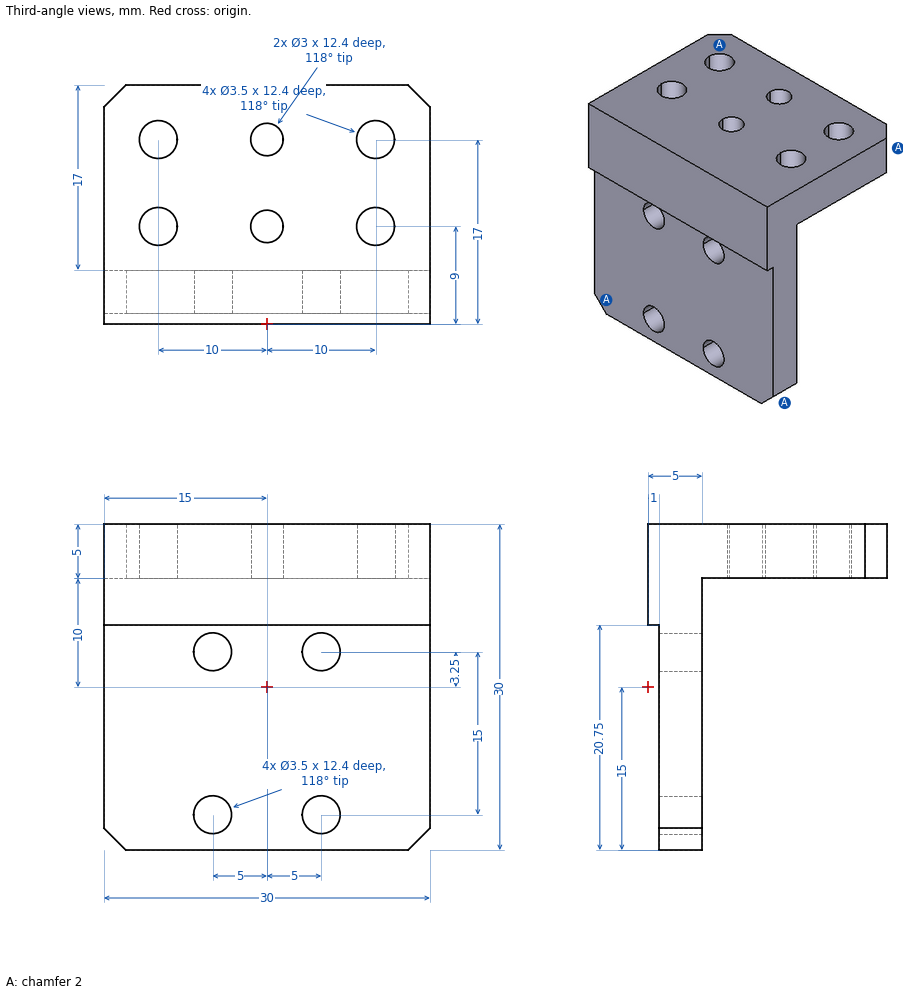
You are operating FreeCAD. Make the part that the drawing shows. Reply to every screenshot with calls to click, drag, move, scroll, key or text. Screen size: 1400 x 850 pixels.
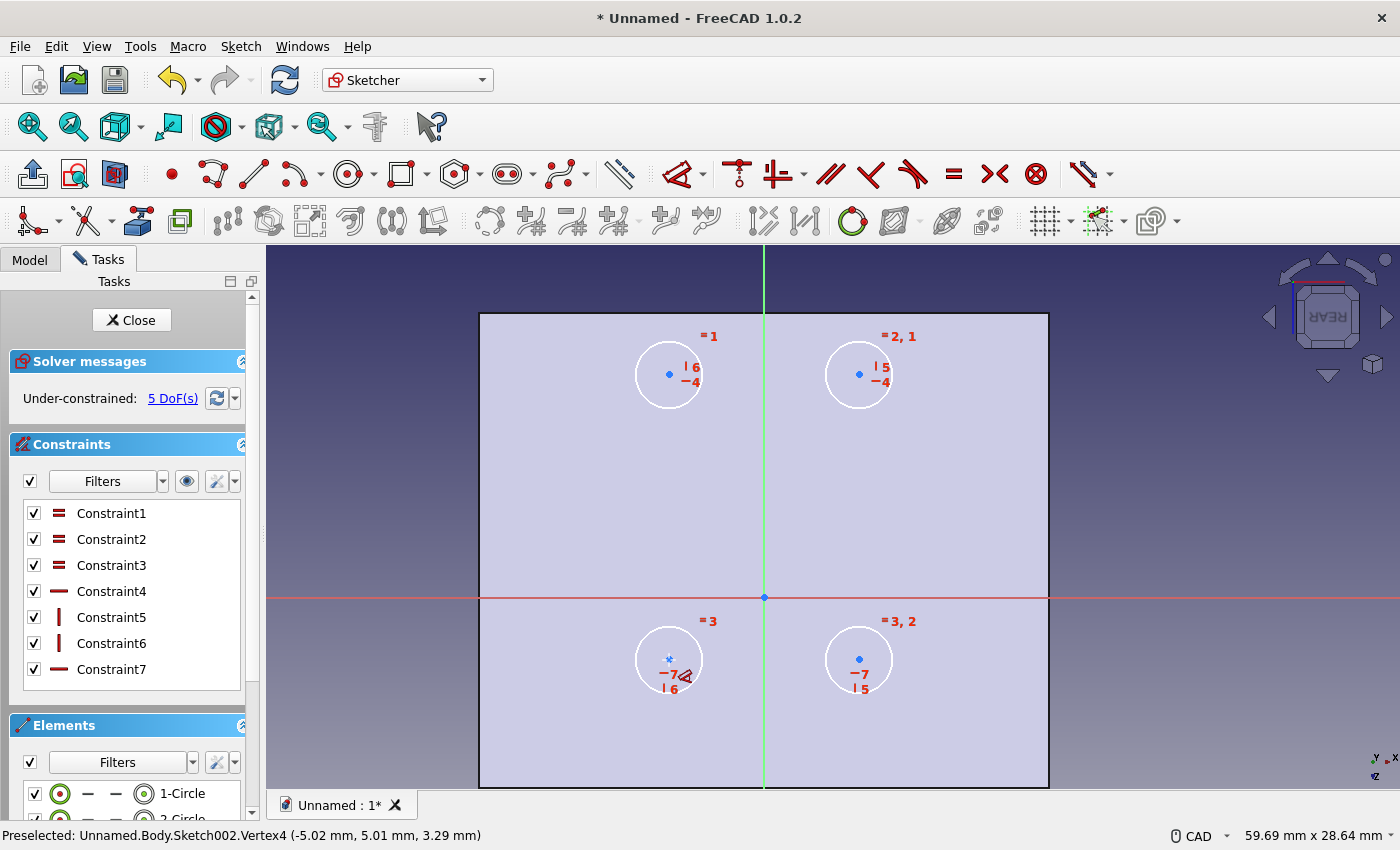
click(692, 351)
click(714, 328)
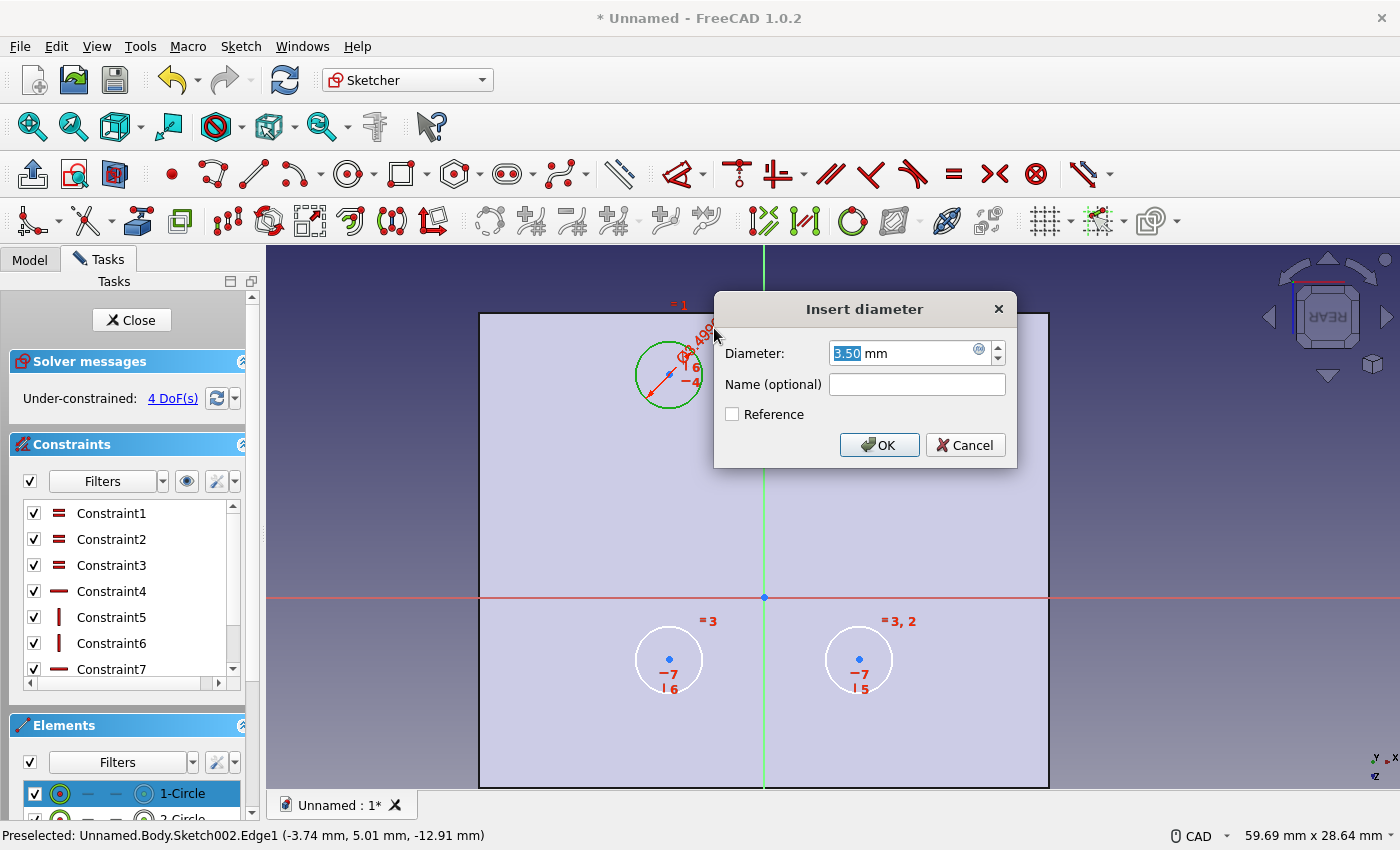
text(3.5)
key(Return)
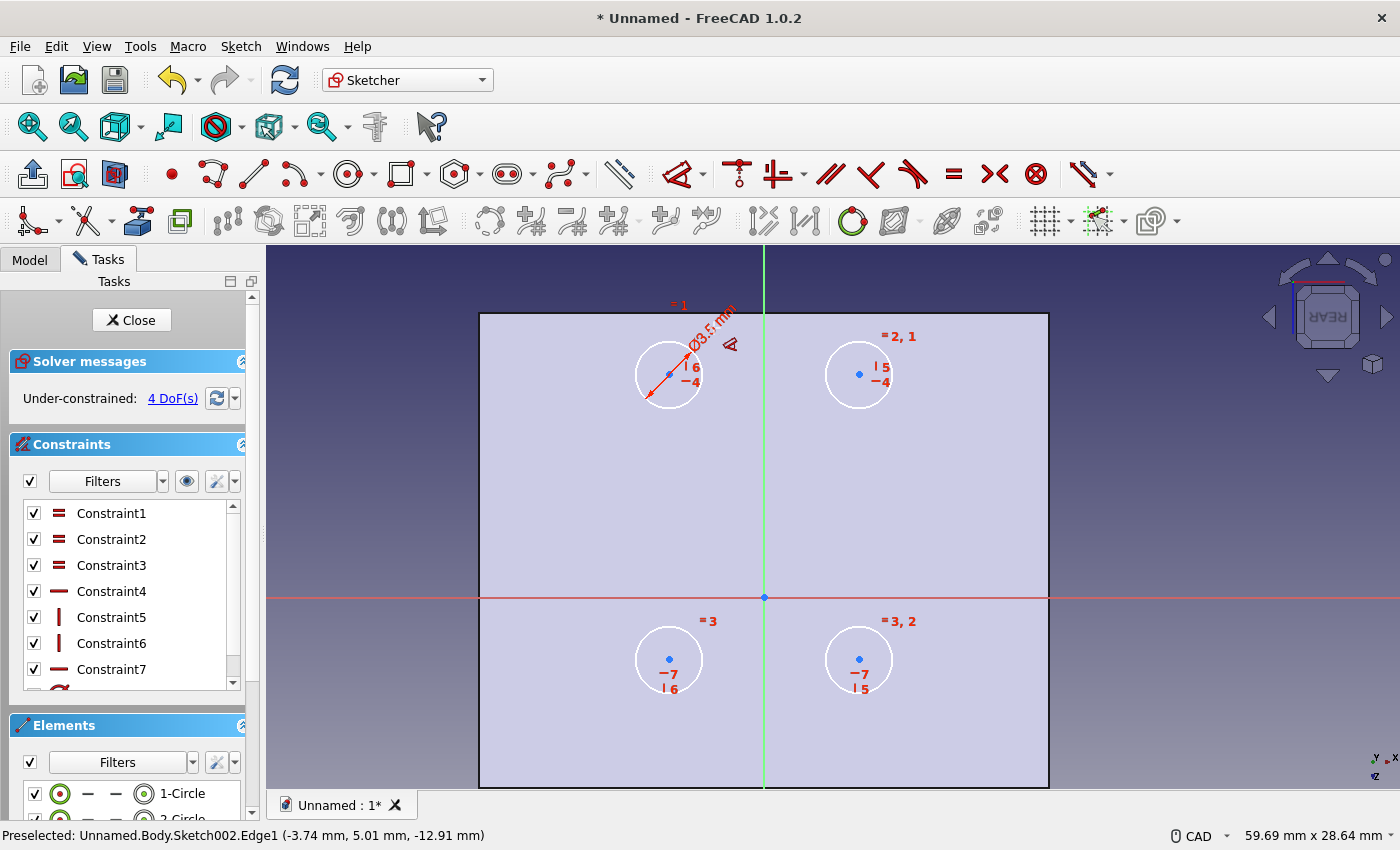
click(669, 375)
click(717, 632)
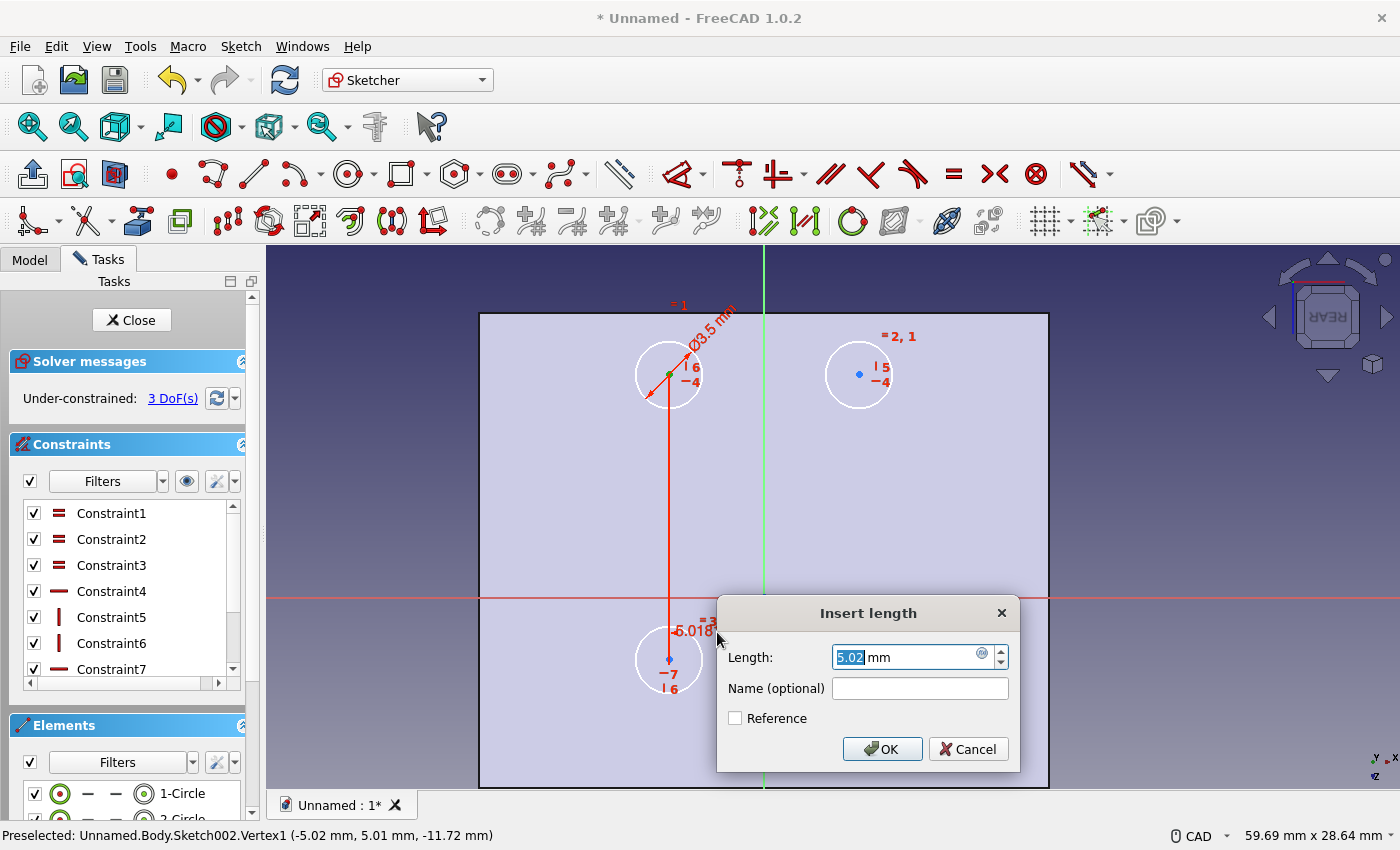
text(5)
key(Return)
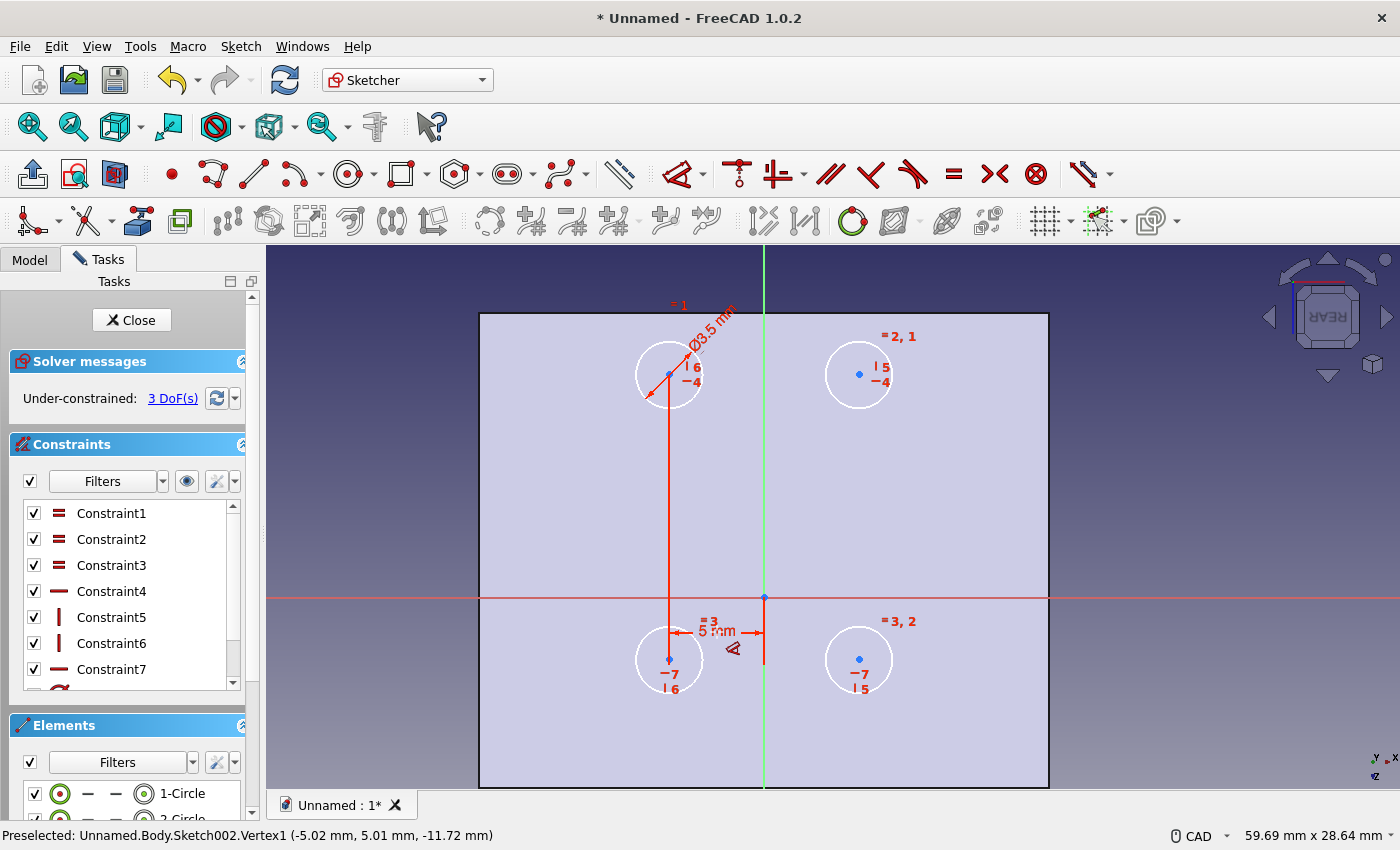
click(859, 375)
click(812, 341)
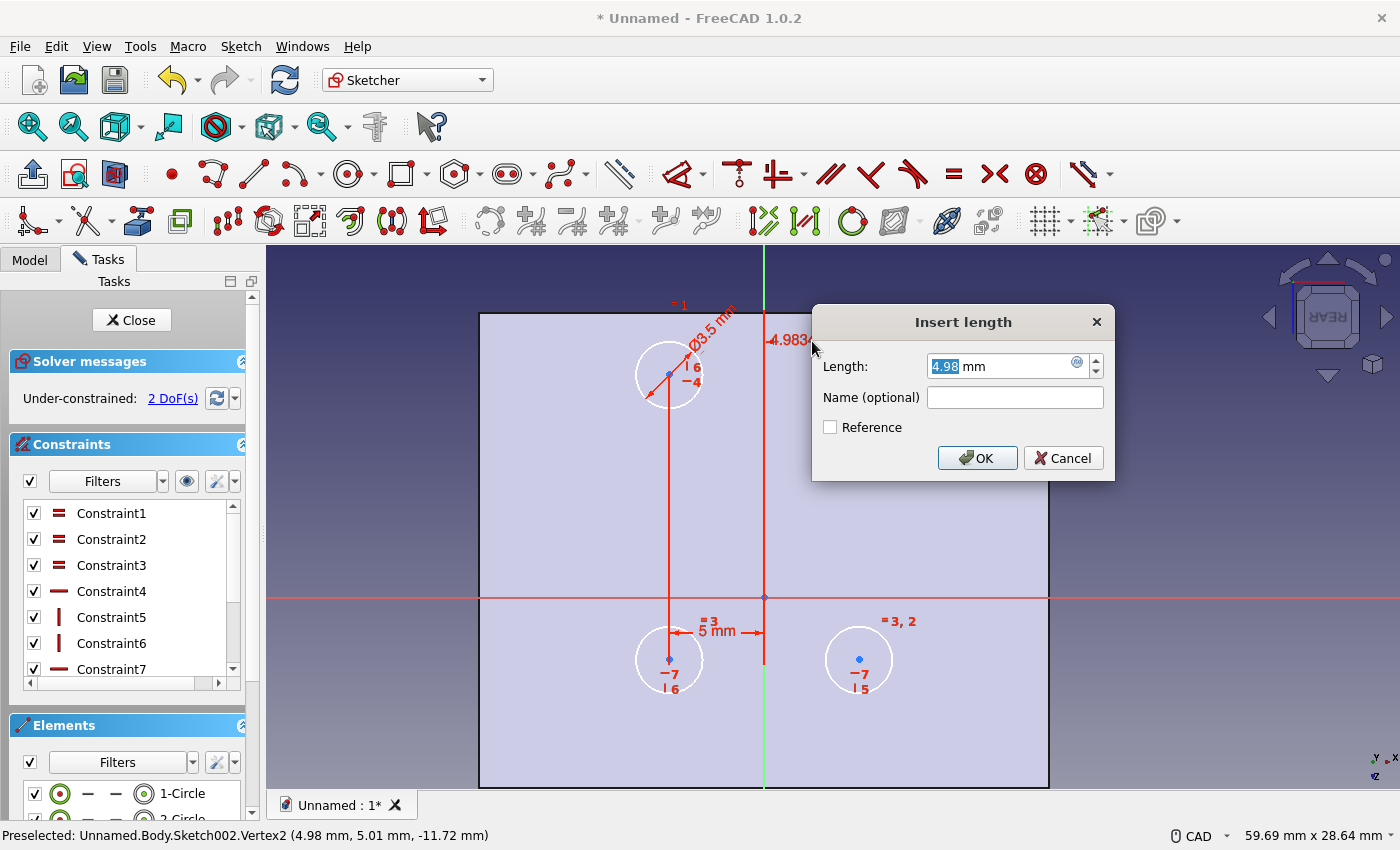
text(5)
key(Return)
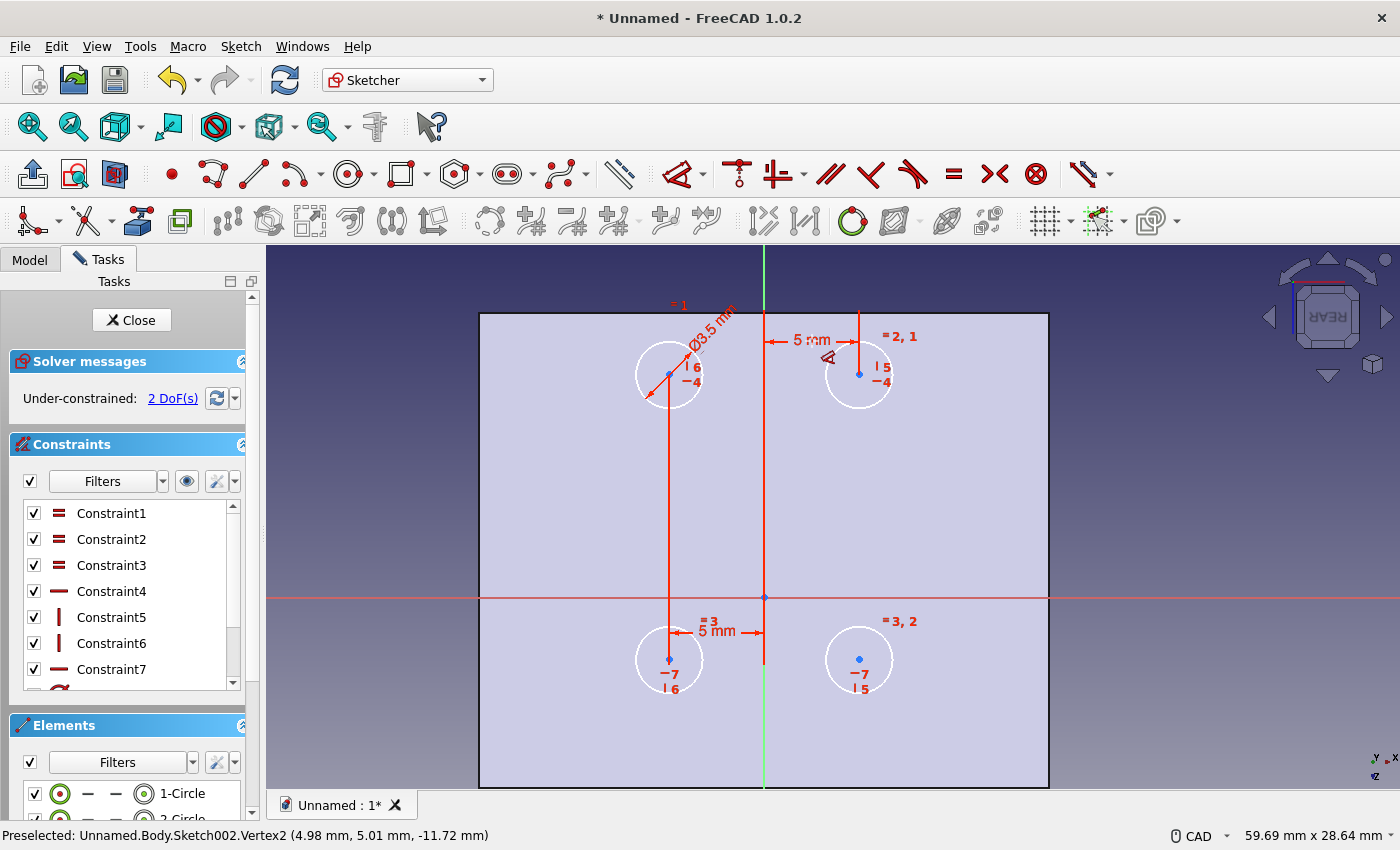
click(859, 375)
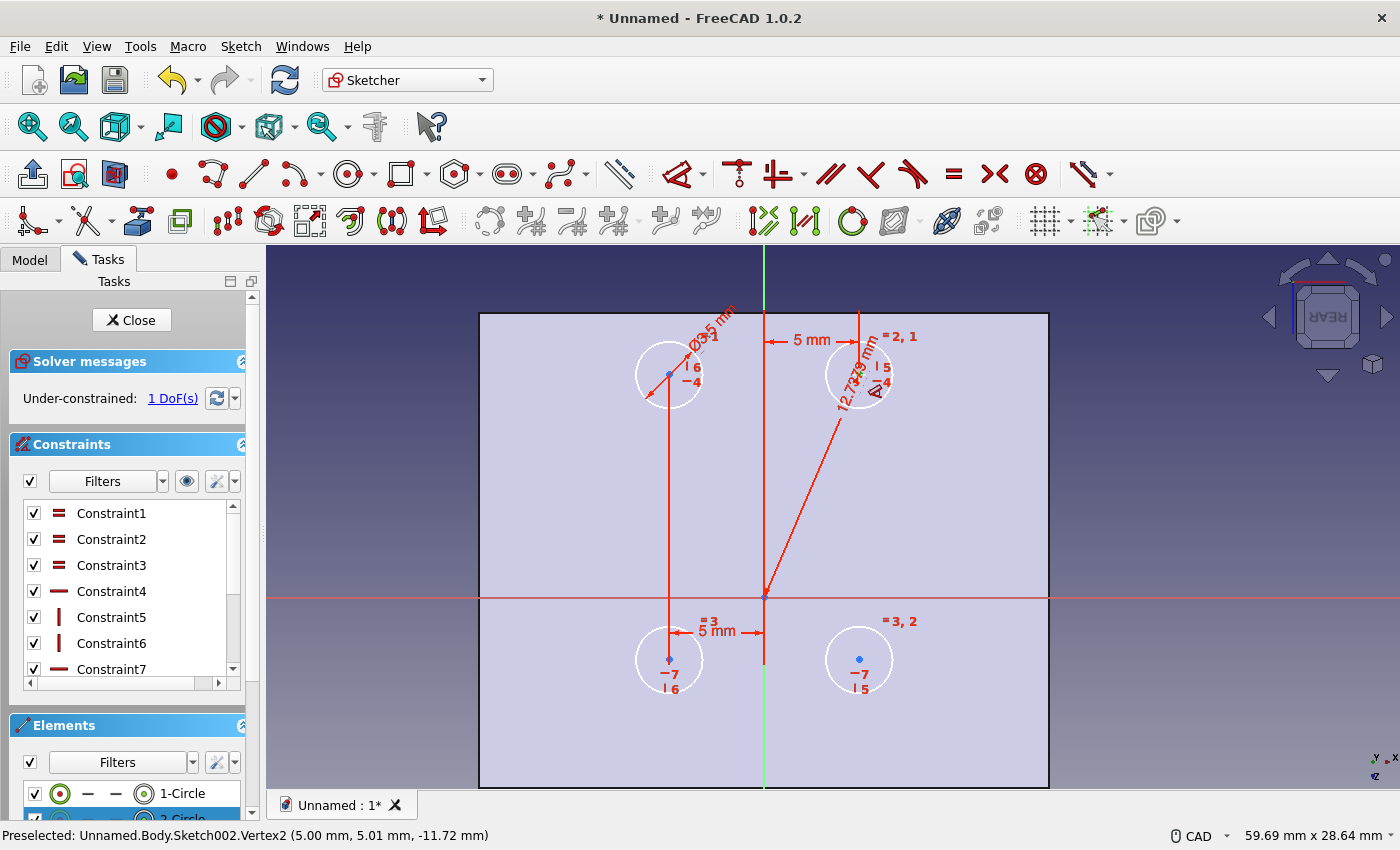
click(859, 660)
click(893, 517)